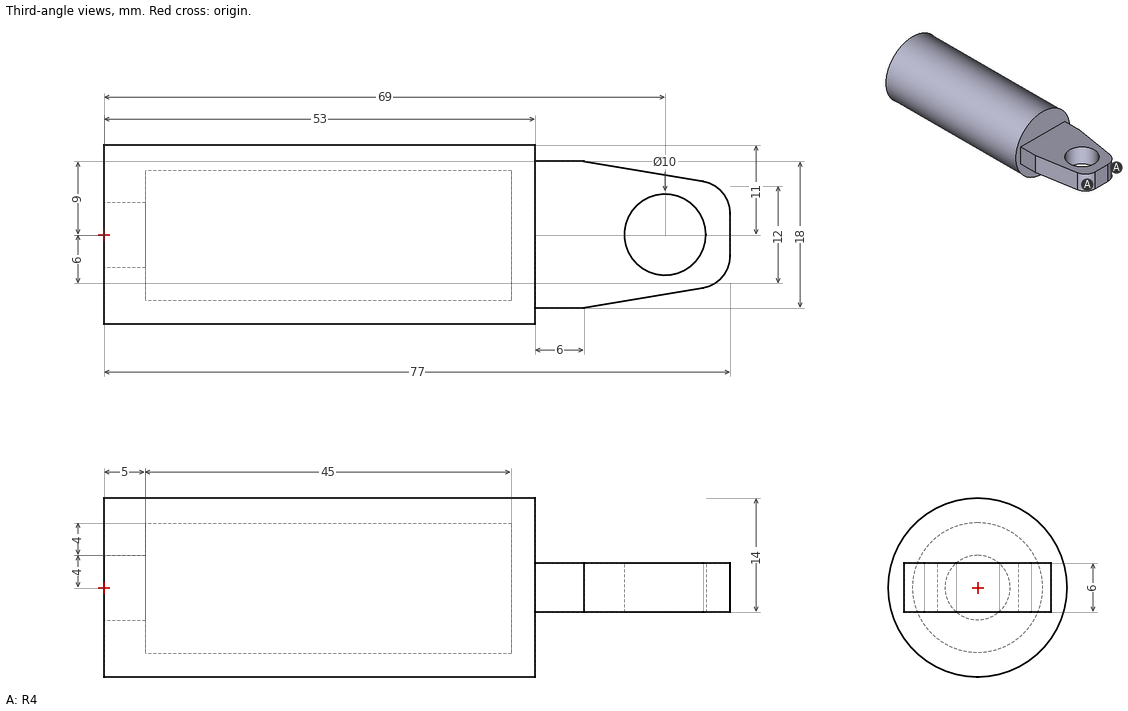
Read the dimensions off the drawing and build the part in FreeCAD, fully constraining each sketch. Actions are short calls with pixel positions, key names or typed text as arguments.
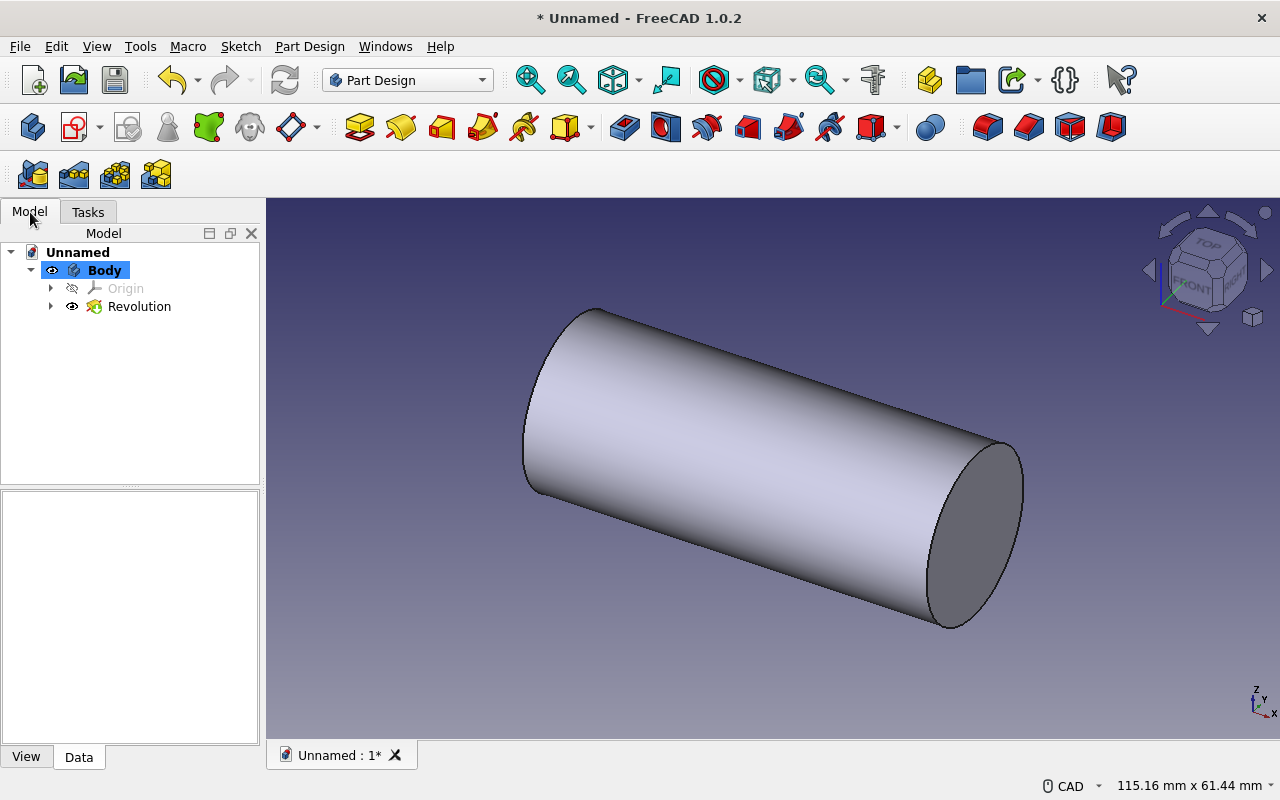
click(51, 288)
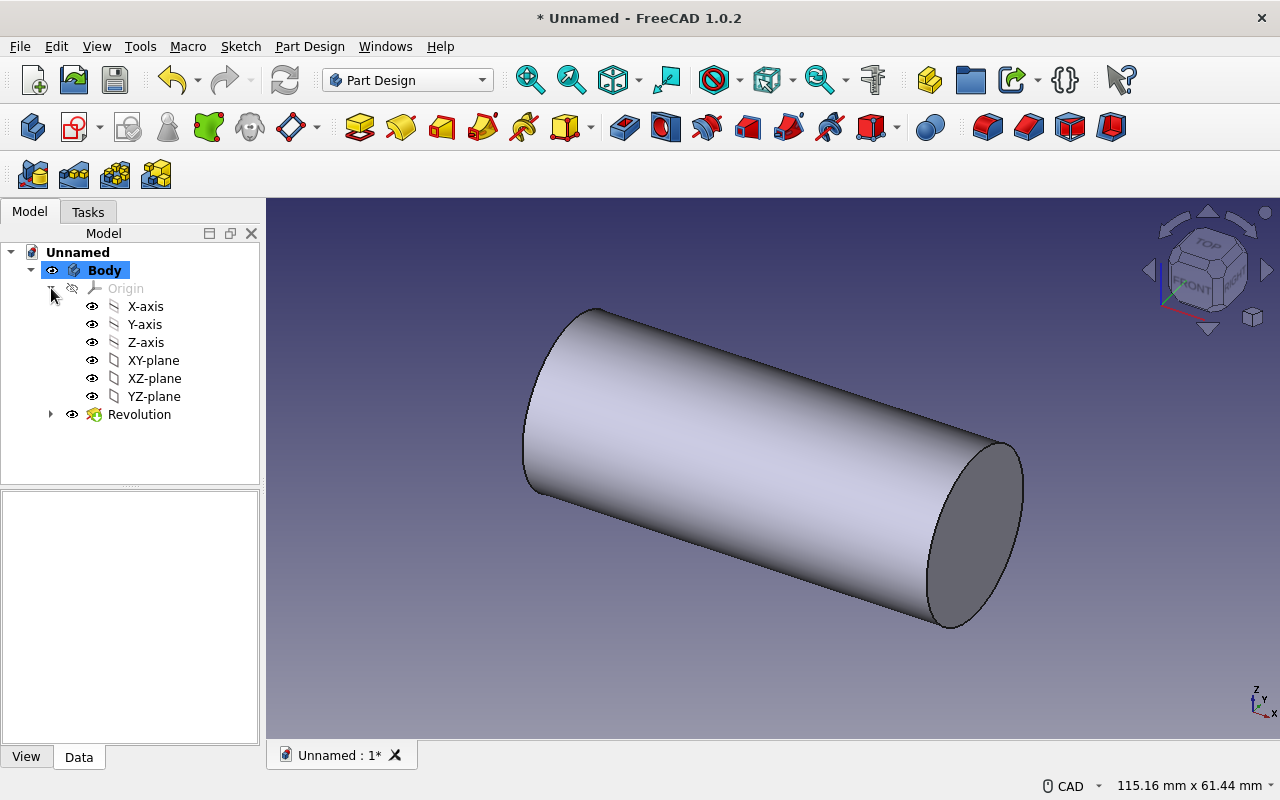
click(137, 360)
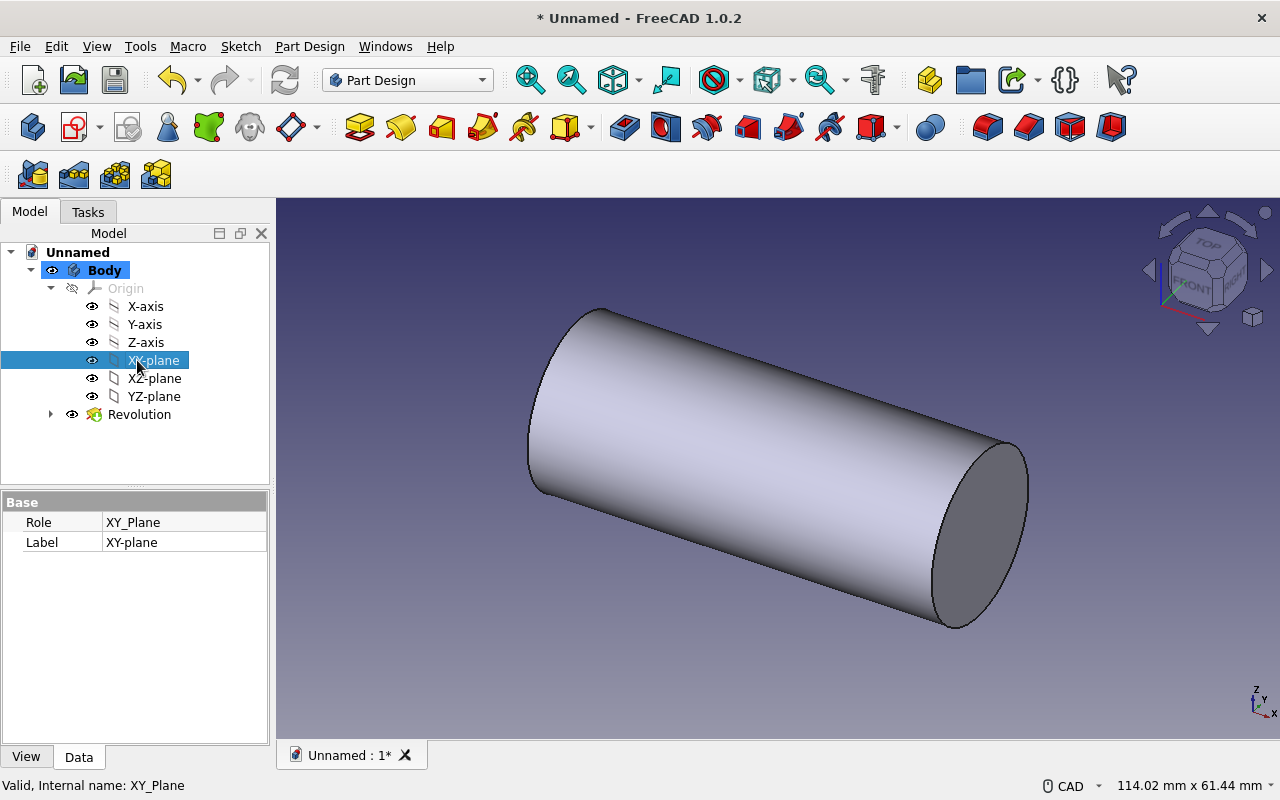
click(290, 128)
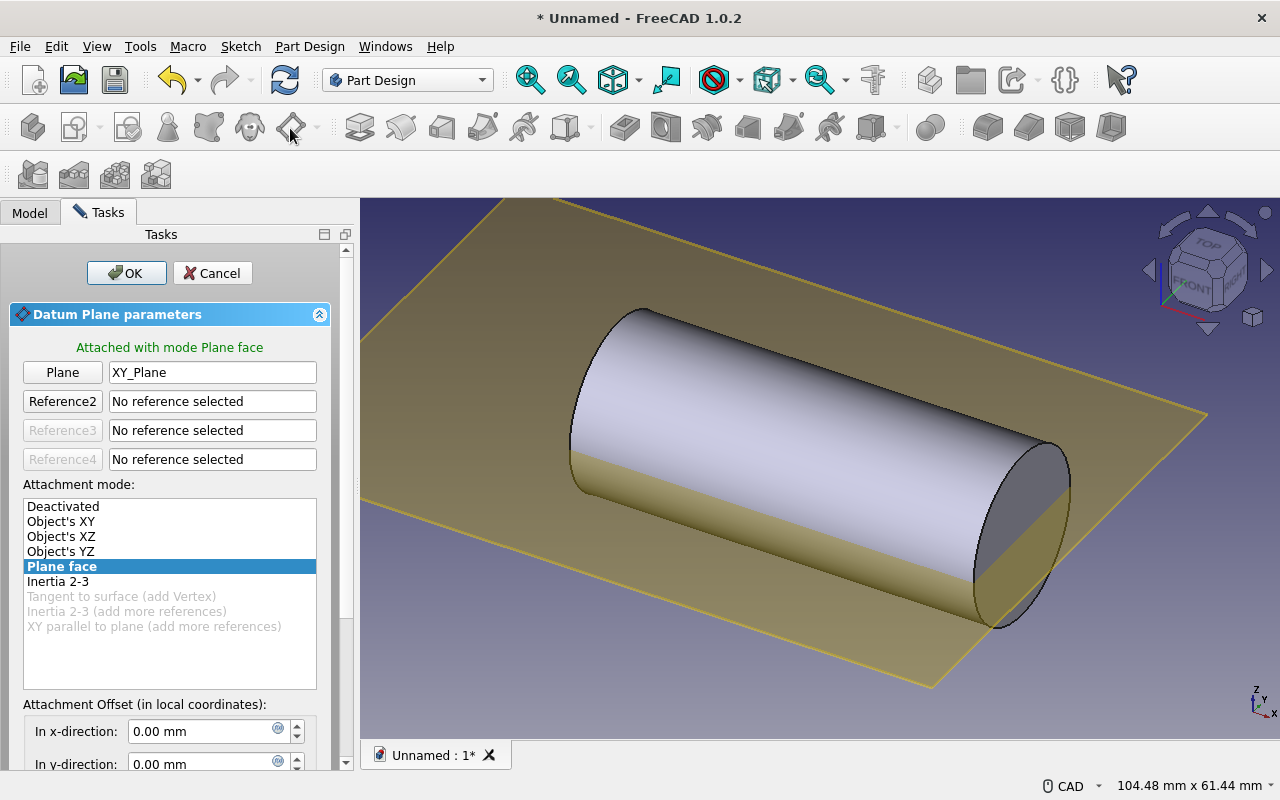
scroll(346, 507, down, 2)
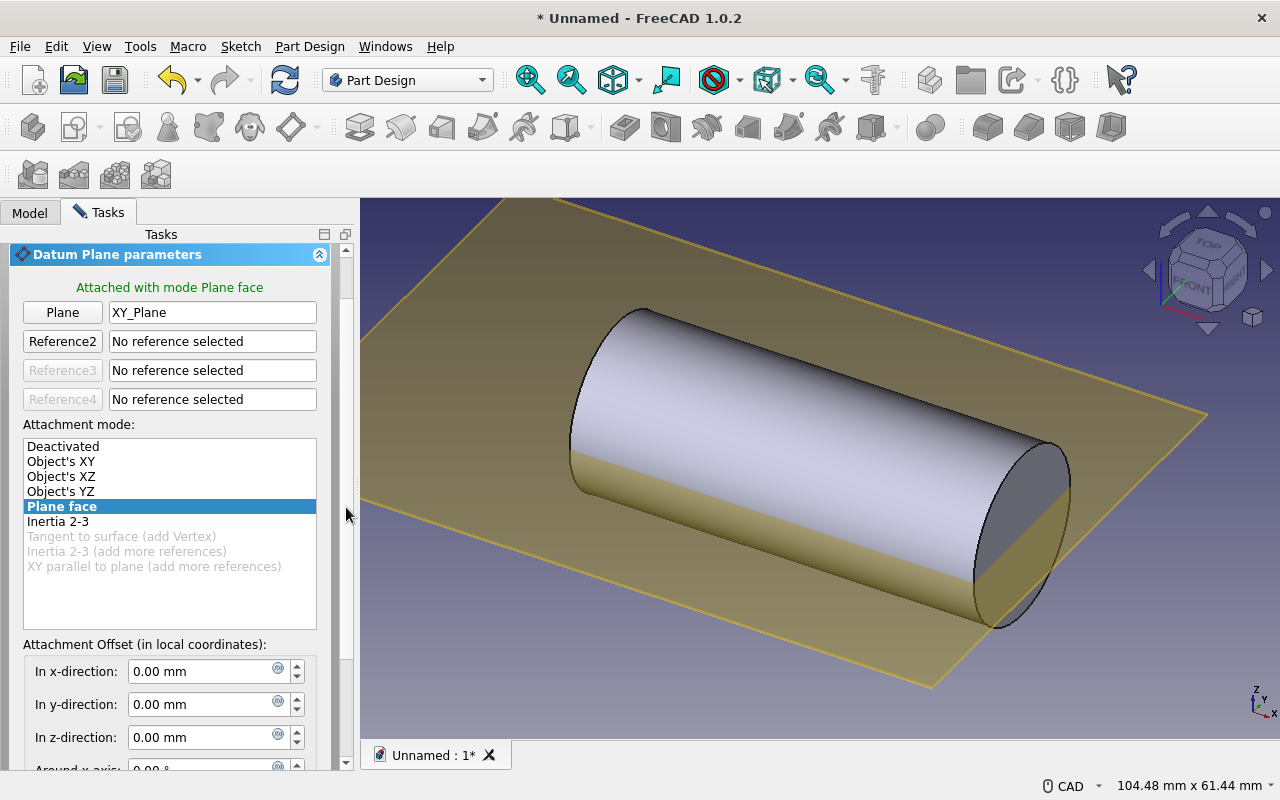
triple_click(210, 678)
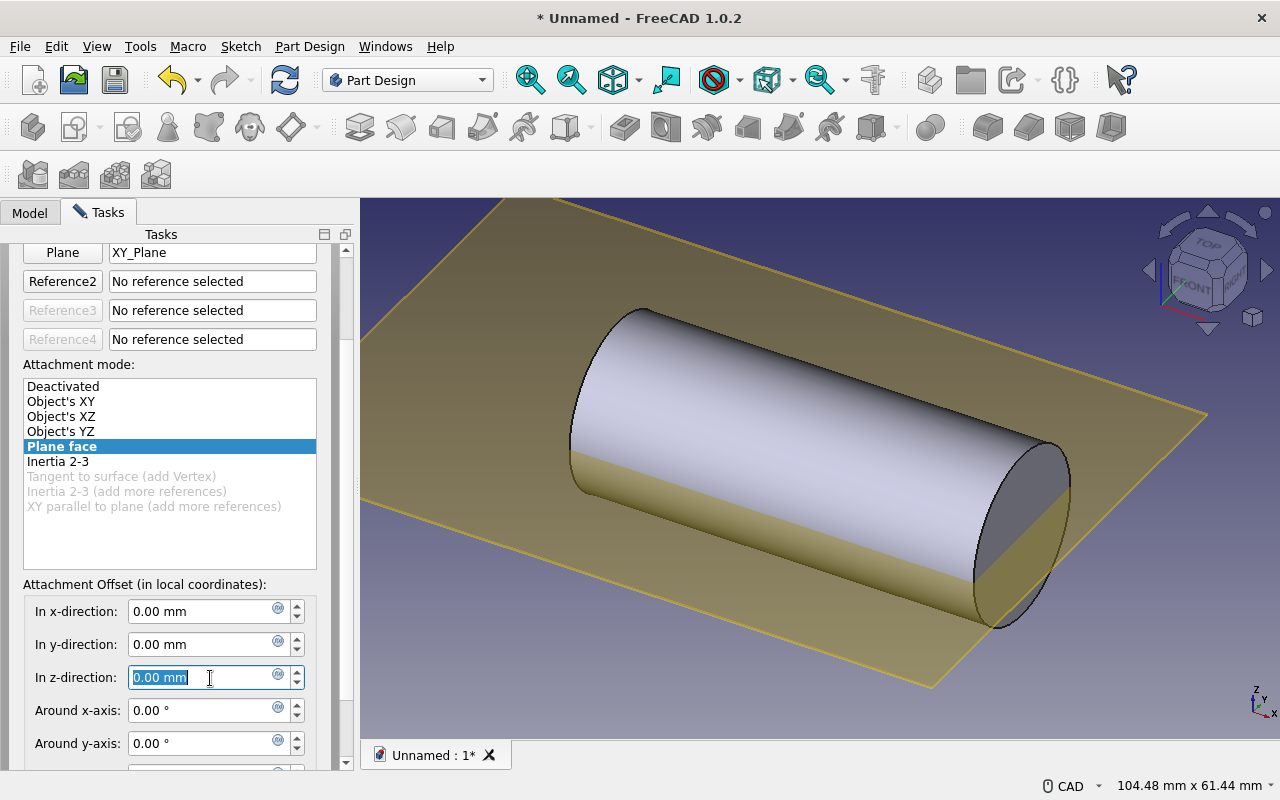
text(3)
key(Tab)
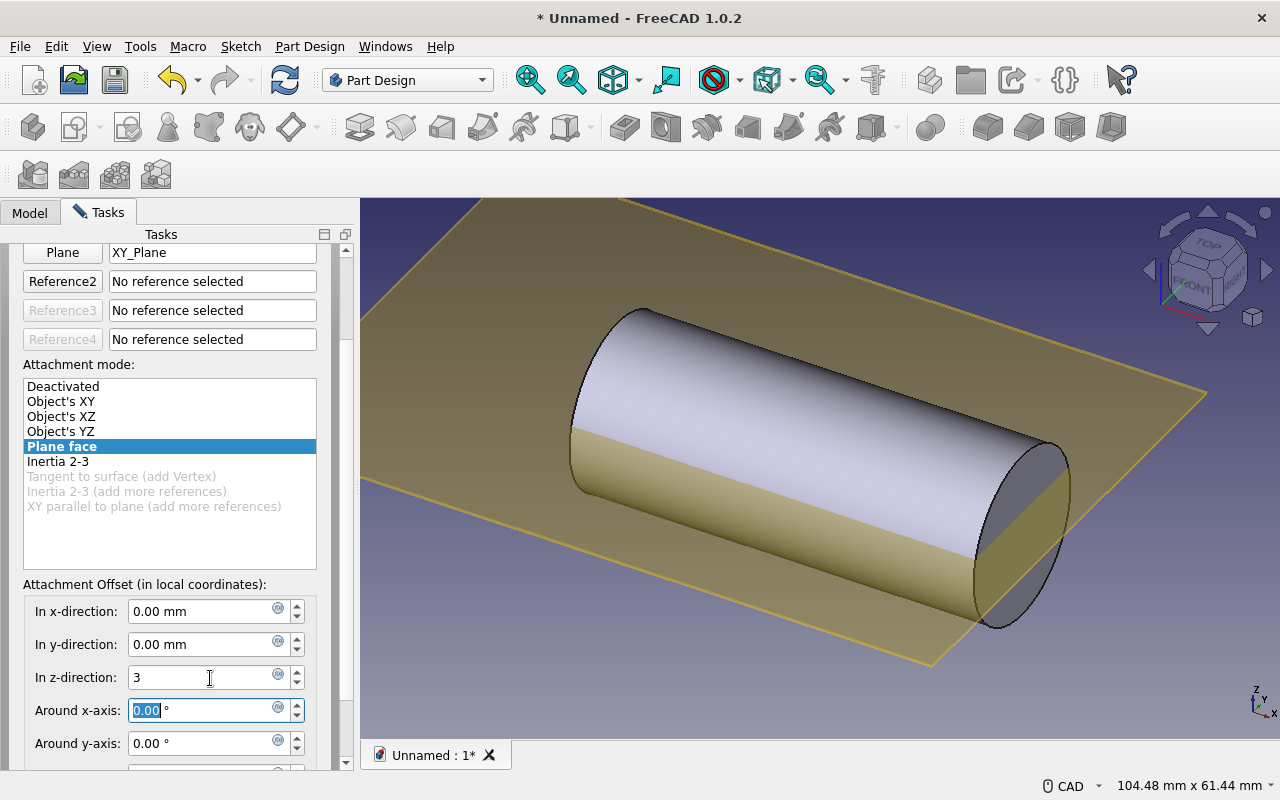
scroll(346, 507, up, 3)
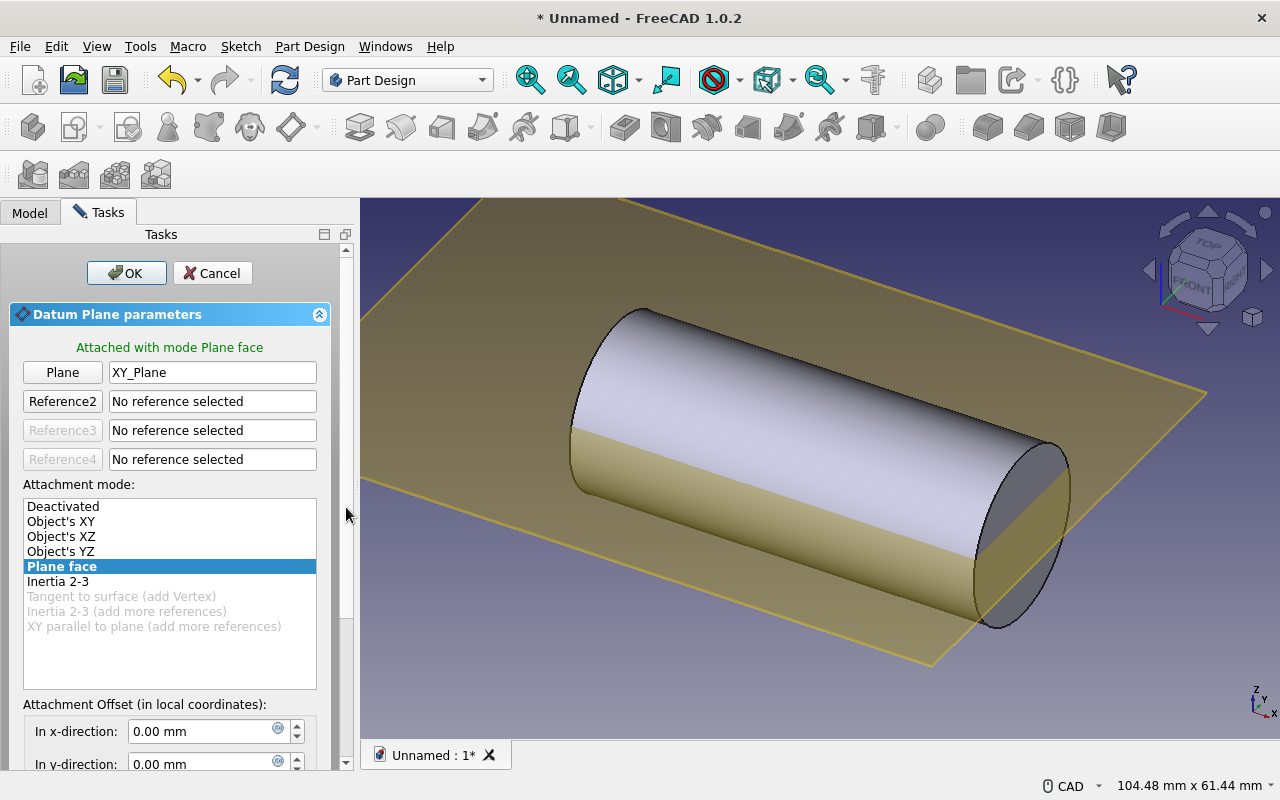
click(127, 273)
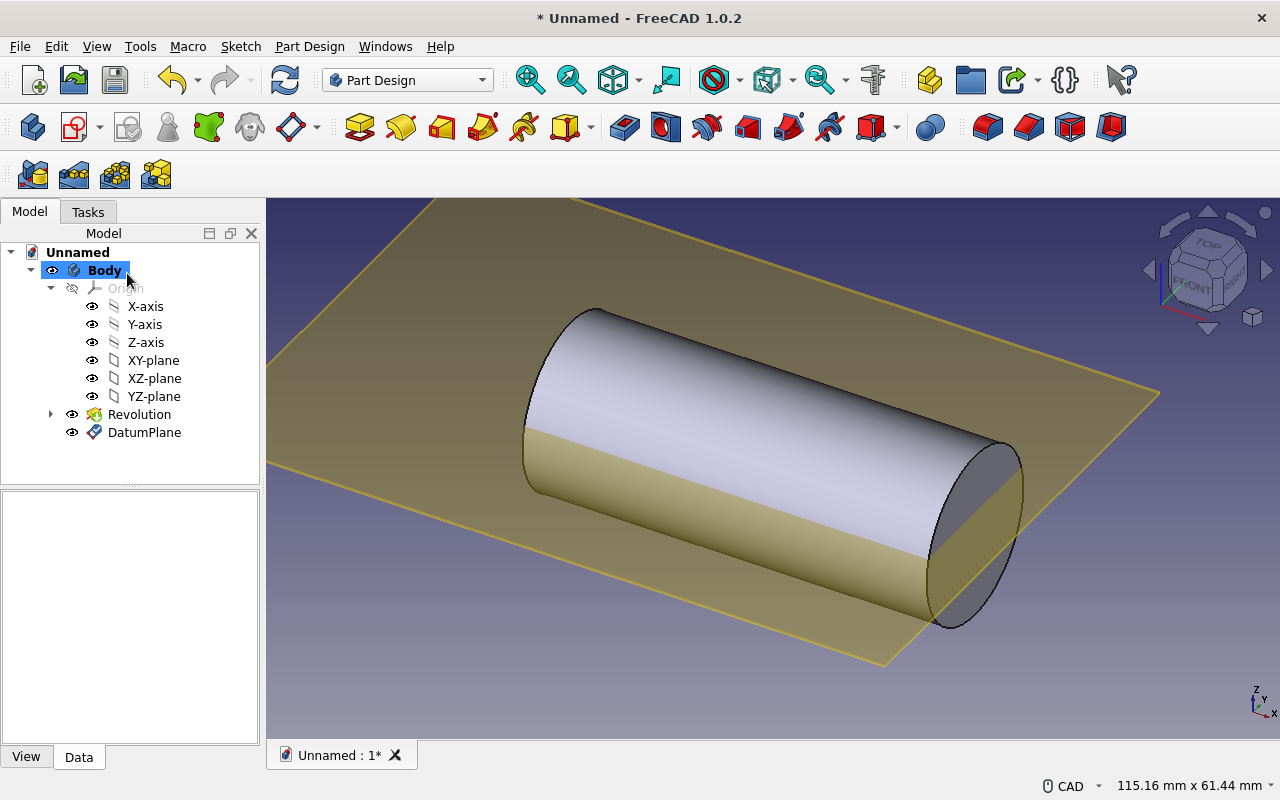
click(117, 432)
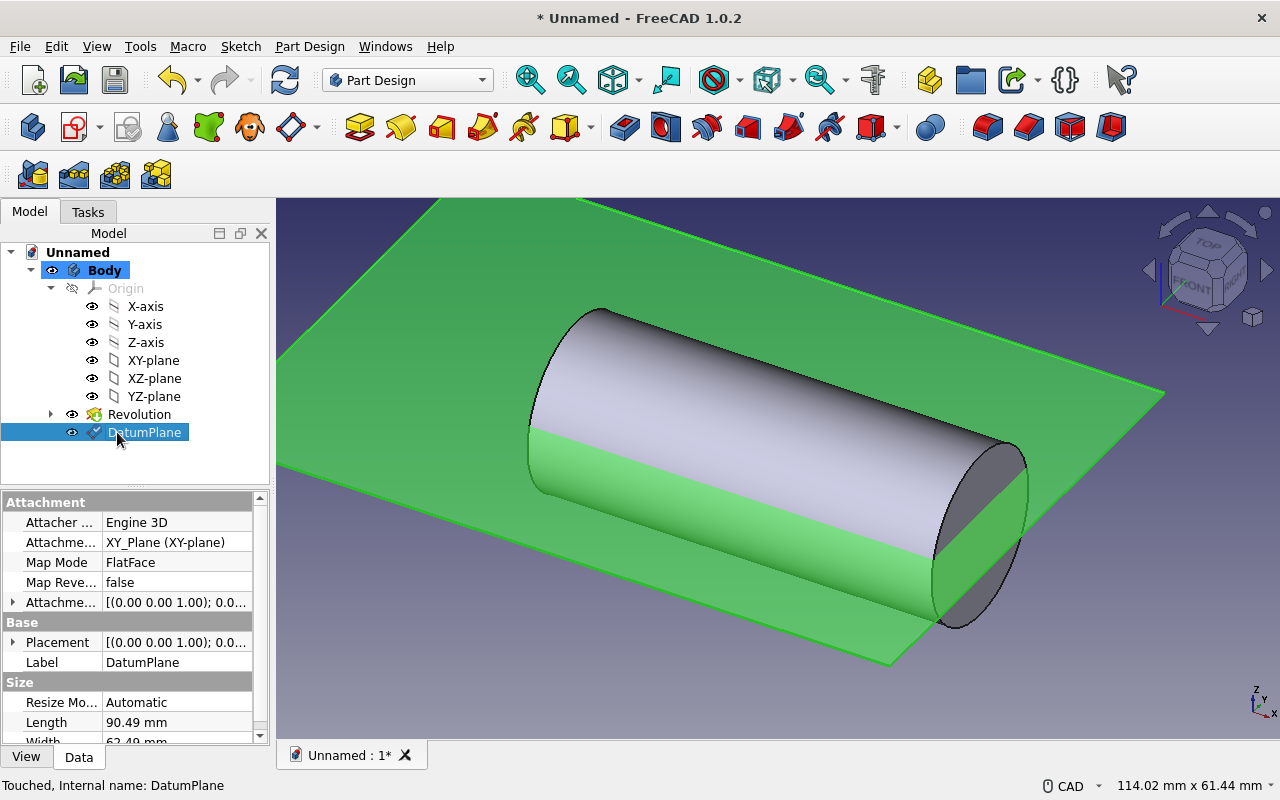
click(74, 128)